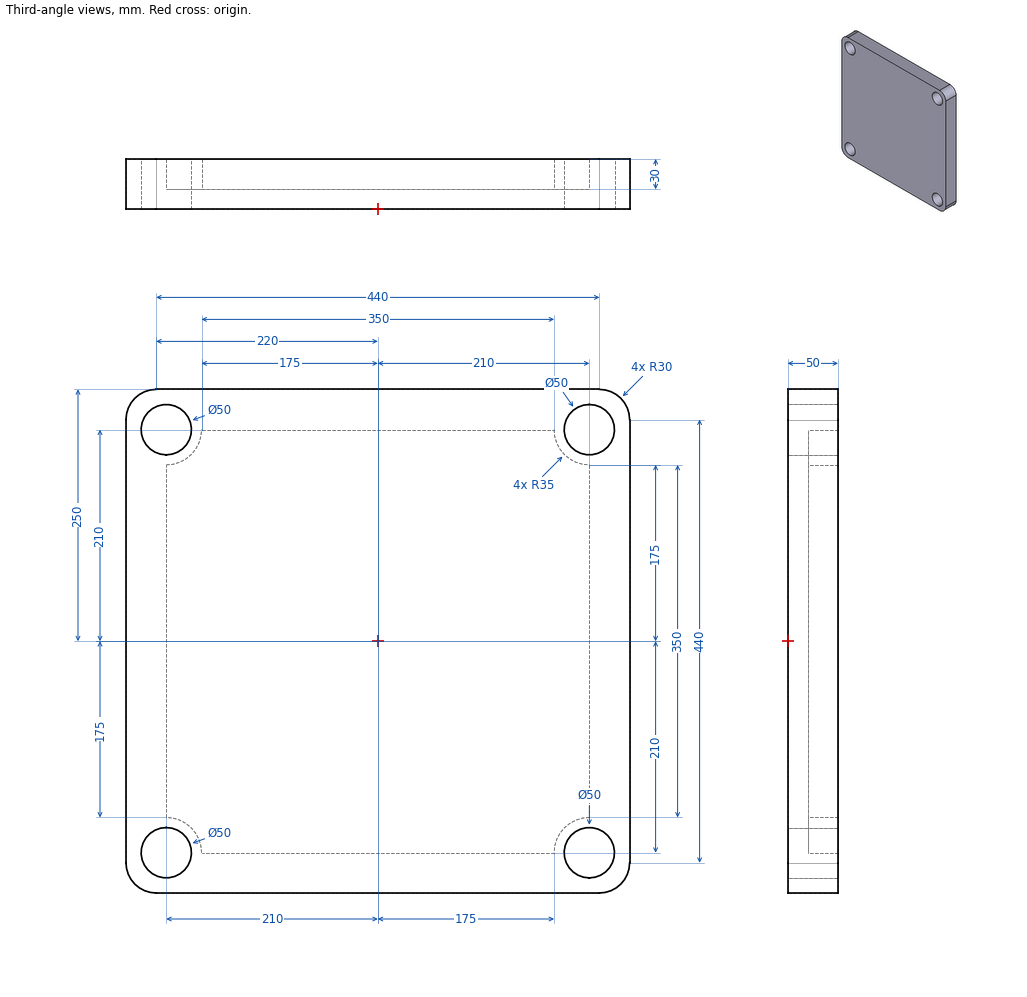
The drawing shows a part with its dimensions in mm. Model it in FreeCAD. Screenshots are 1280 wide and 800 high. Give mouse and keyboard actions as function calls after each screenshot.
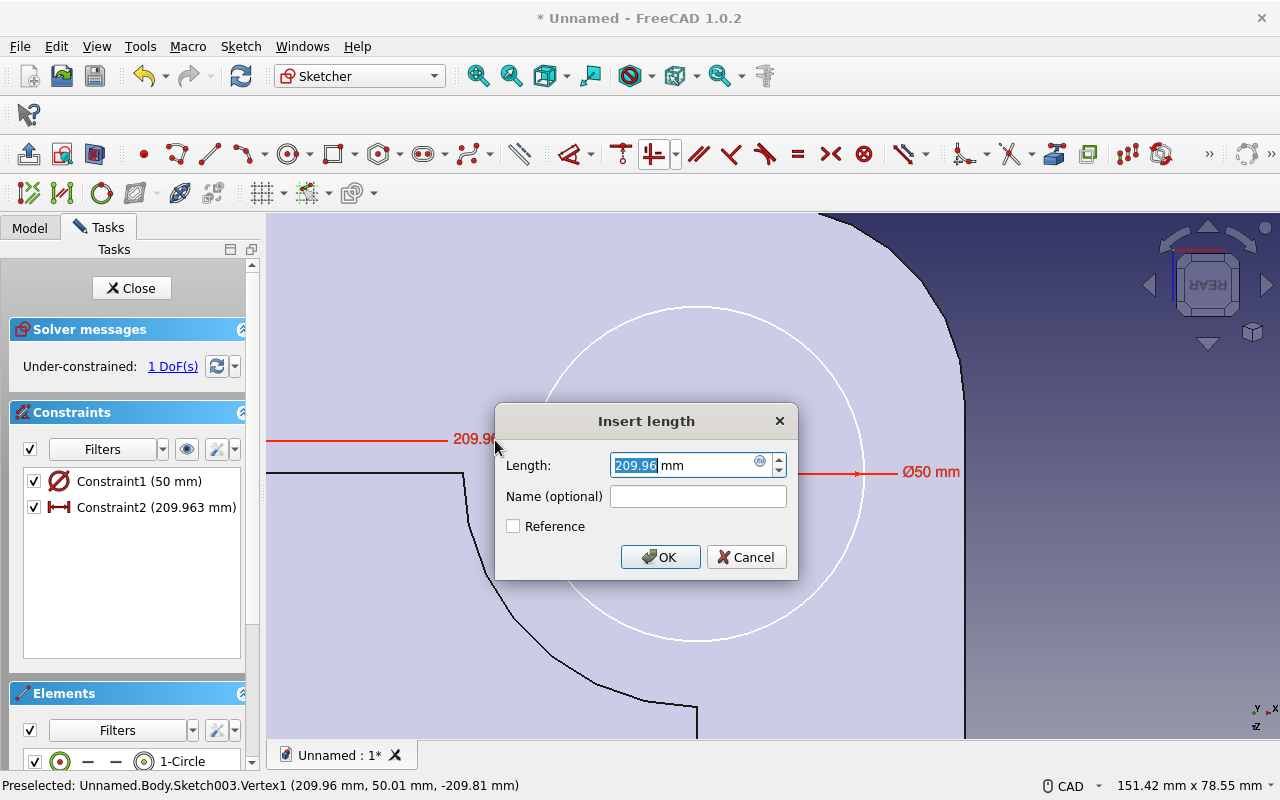
text(210)
key(Return)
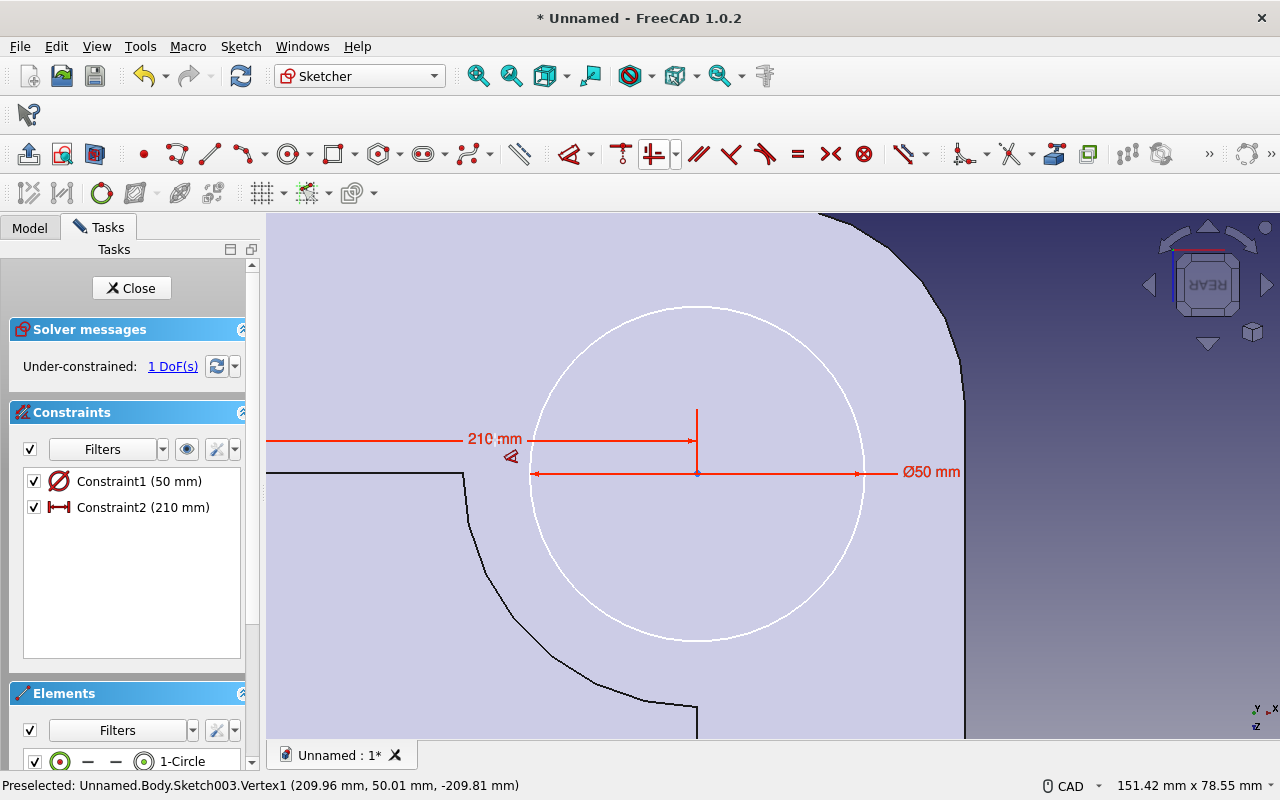
click(697, 474)
click(731, 592)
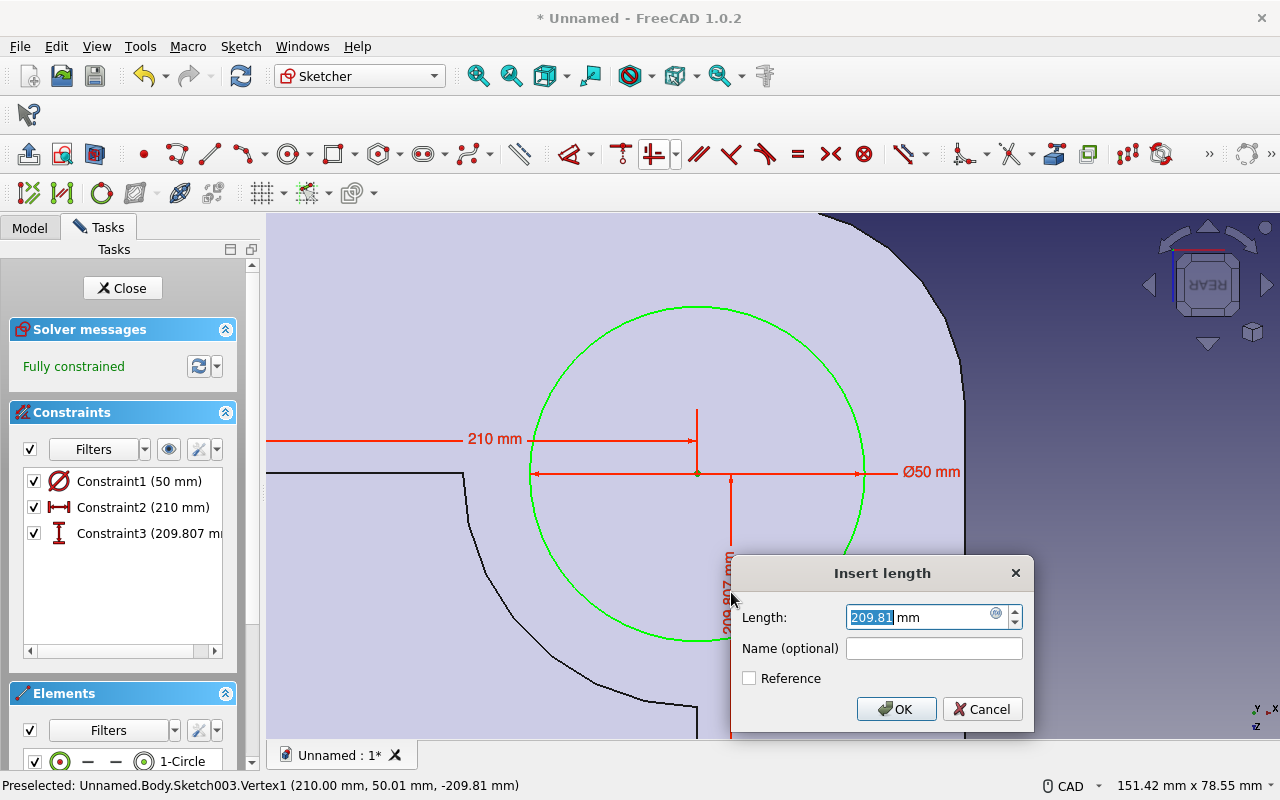
text(210)
key(Return)
key(Escape)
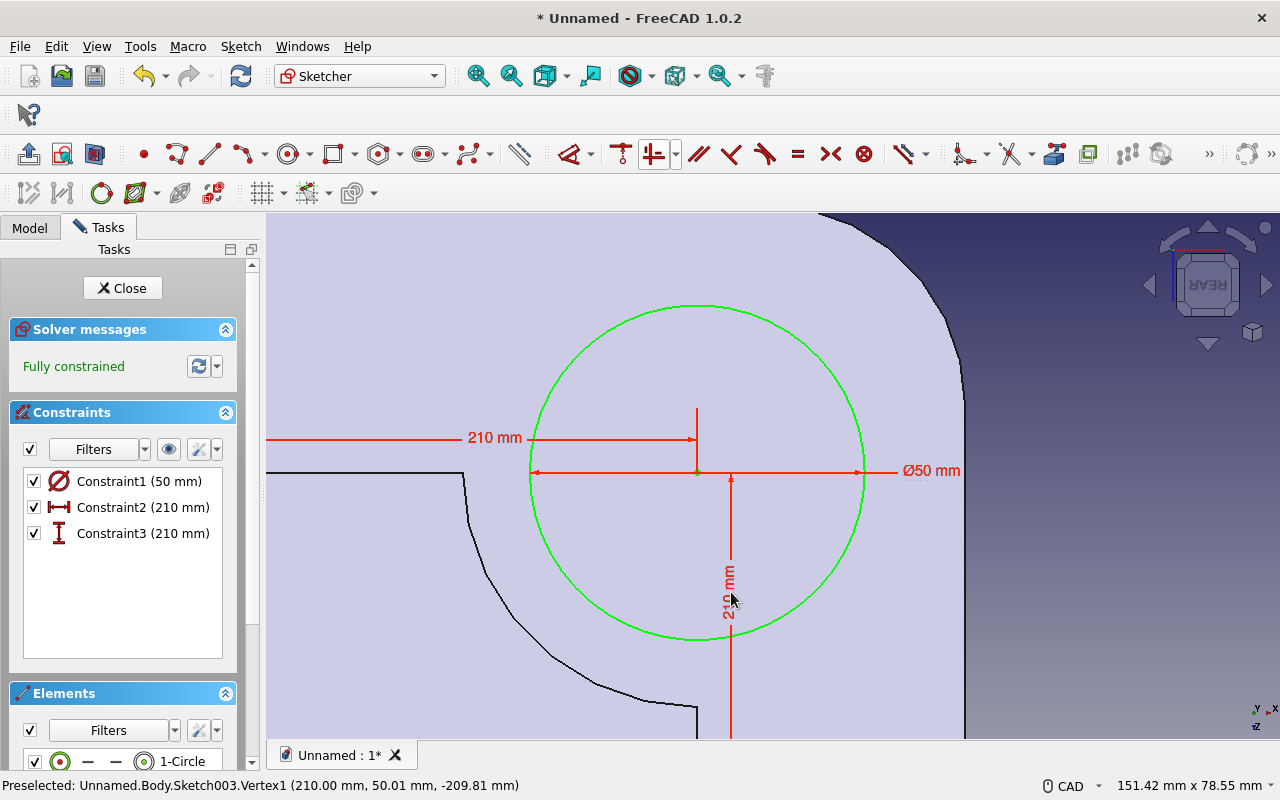
click(123, 288)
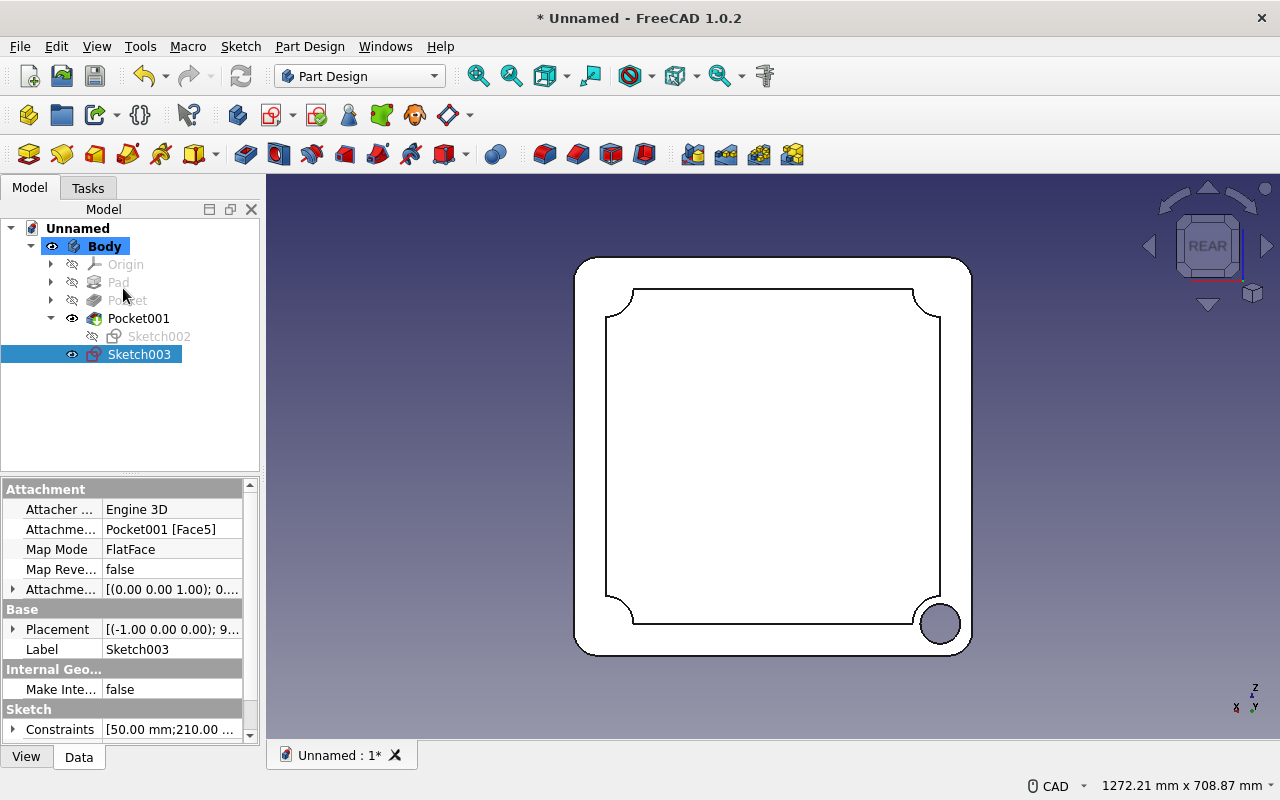
click(246, 154)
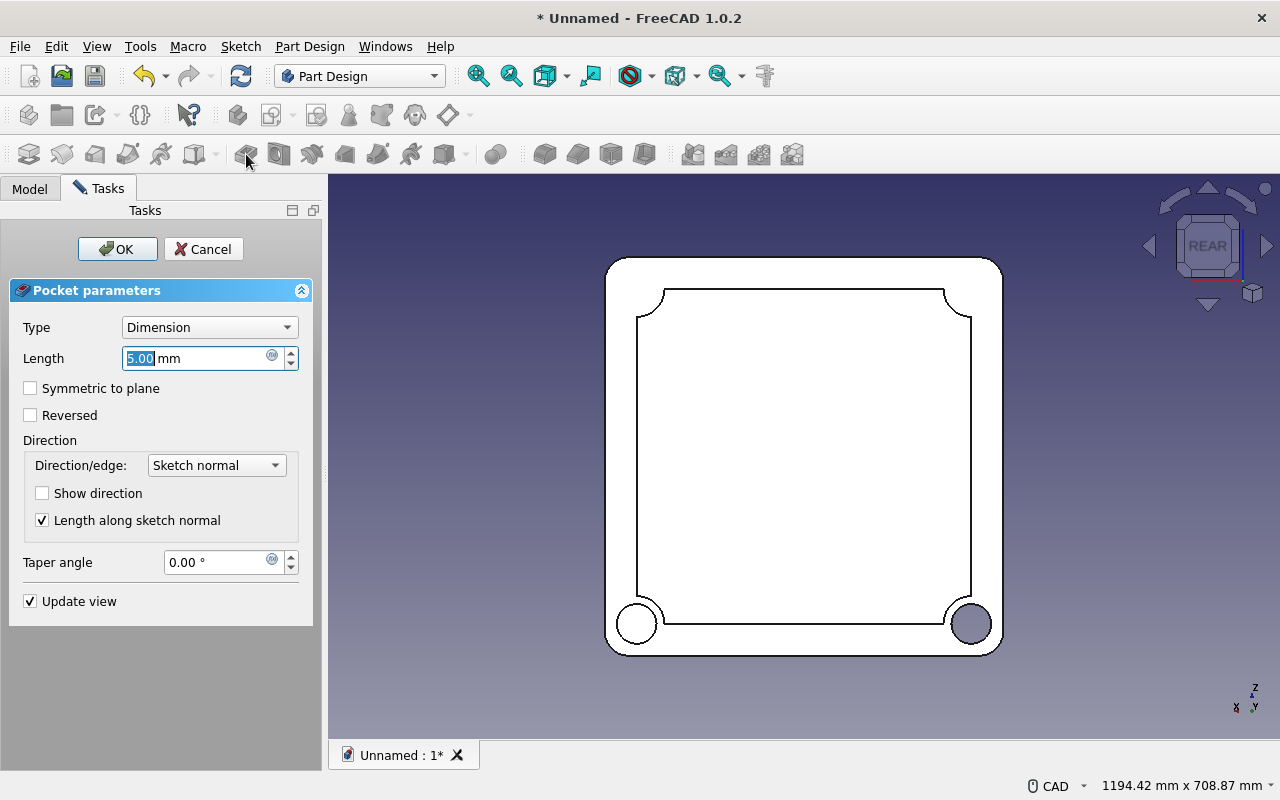
click(210, 328)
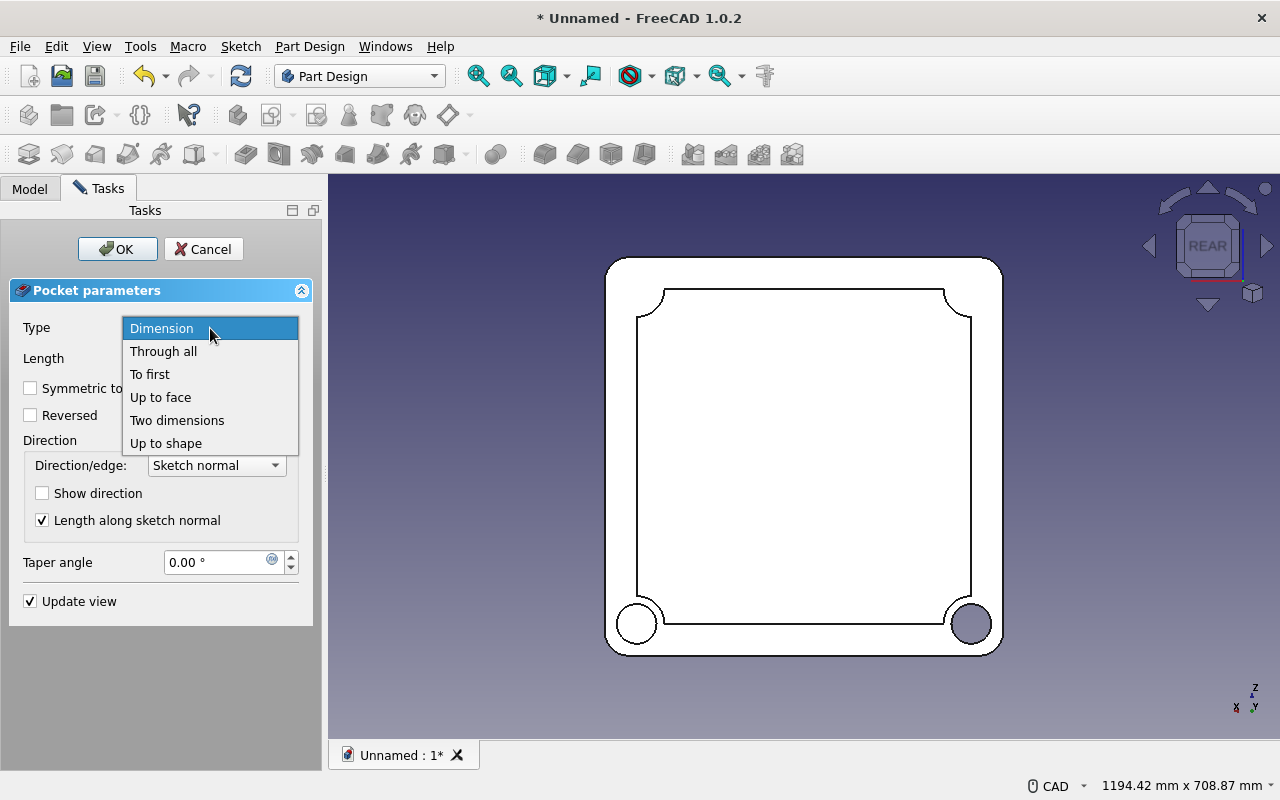
click(208, 374)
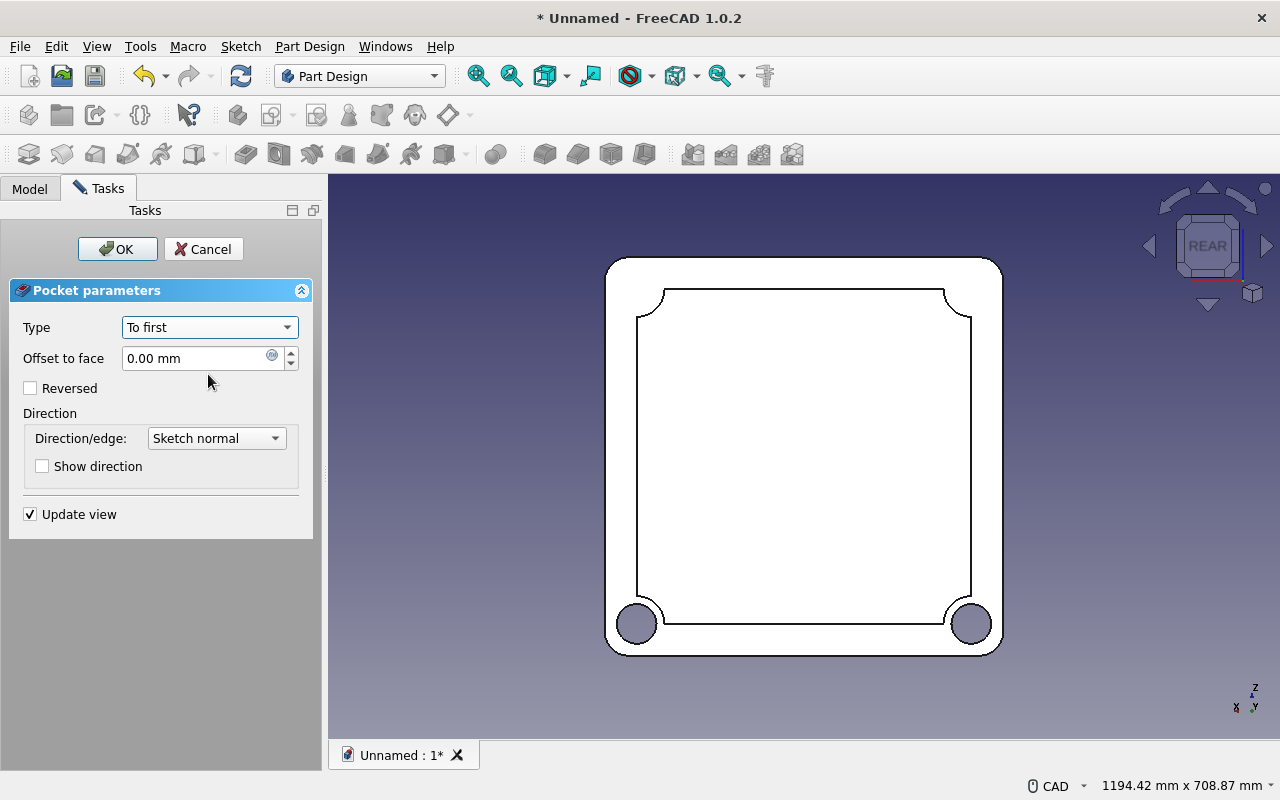
click(118, 249)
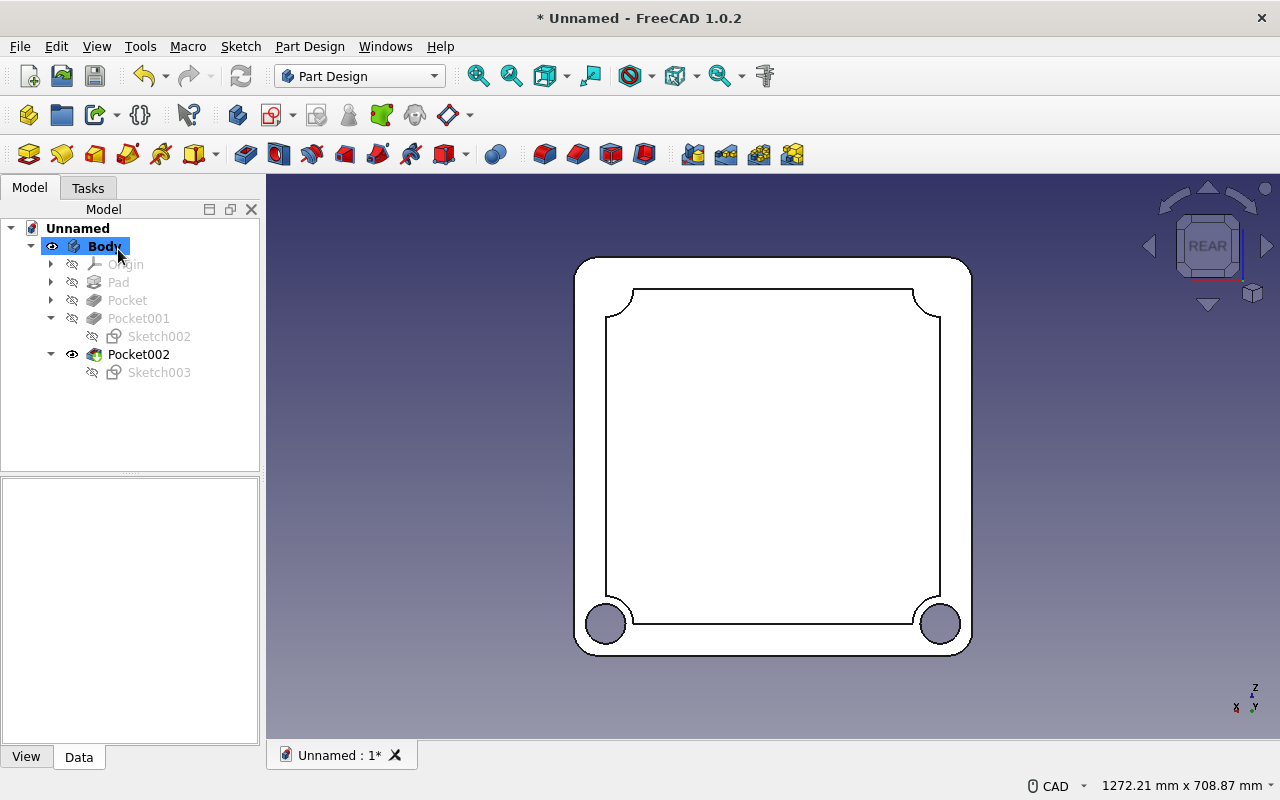
click(602, 285)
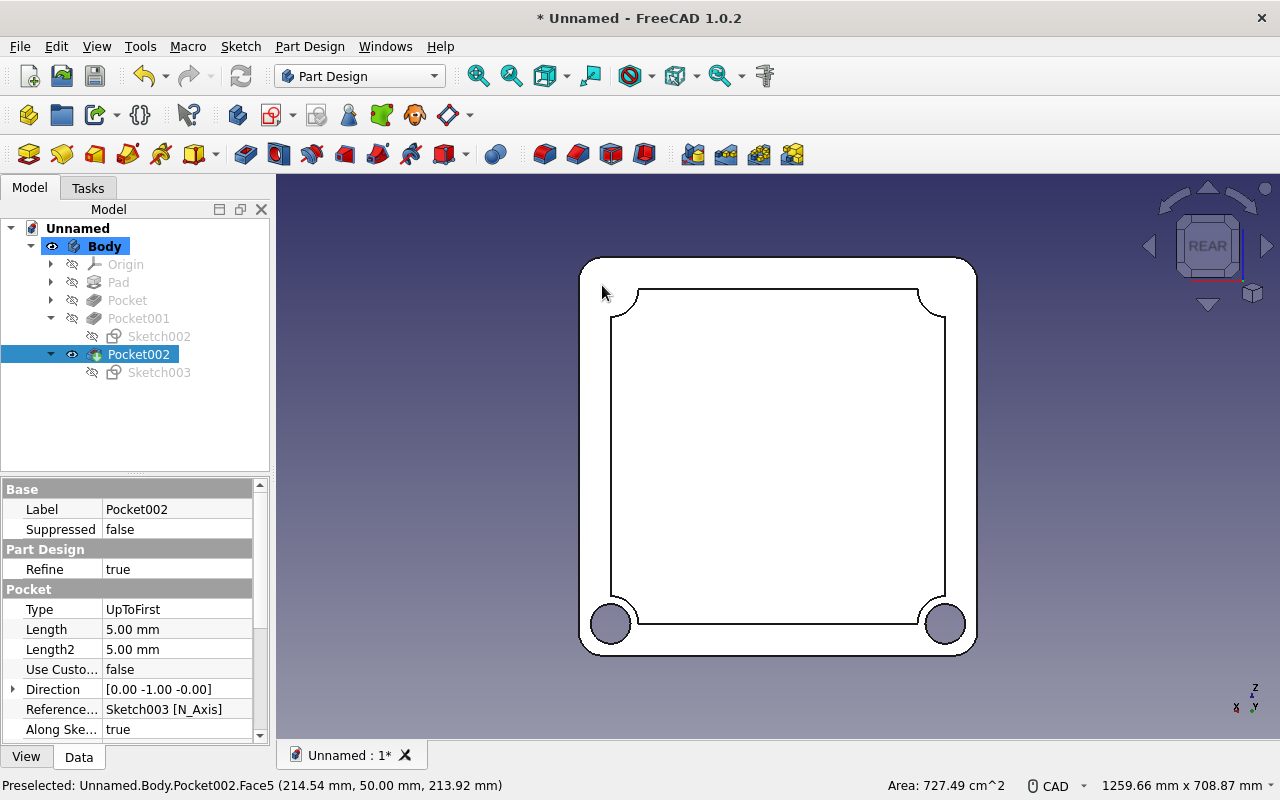
click(270, 116)